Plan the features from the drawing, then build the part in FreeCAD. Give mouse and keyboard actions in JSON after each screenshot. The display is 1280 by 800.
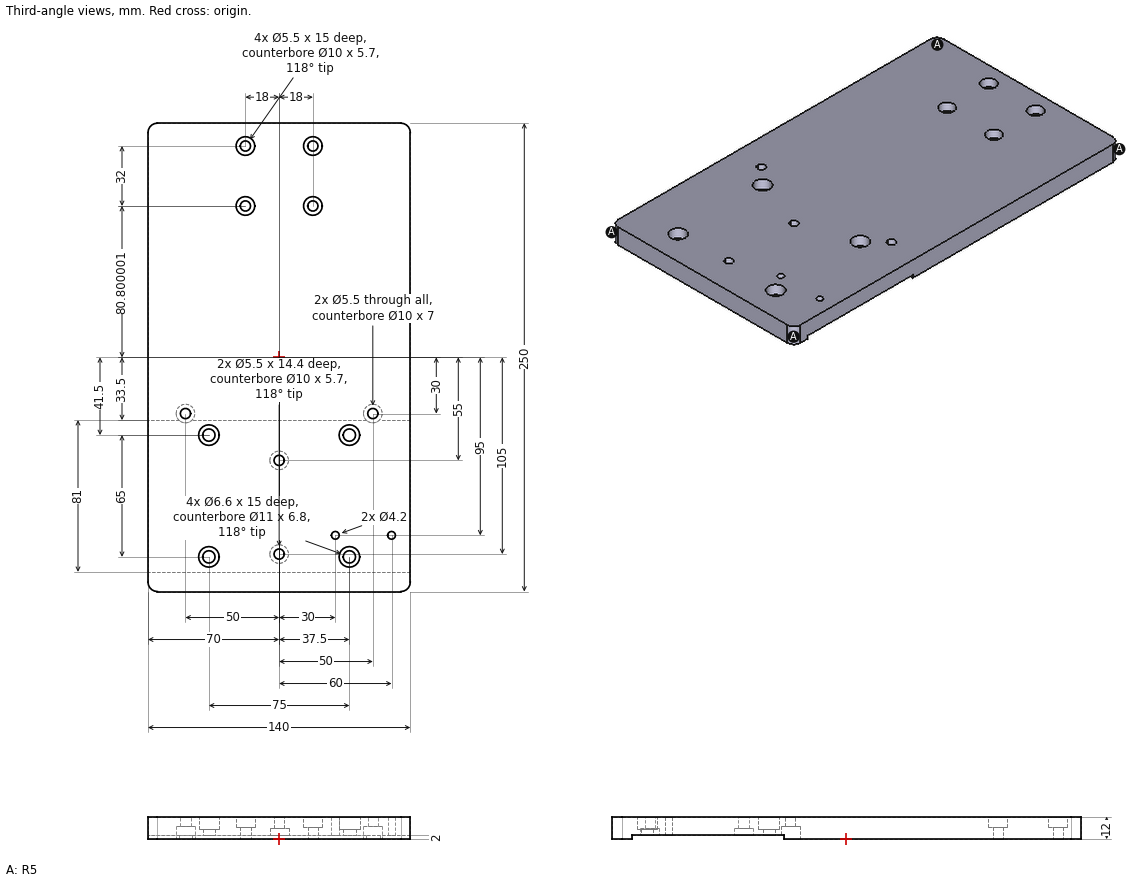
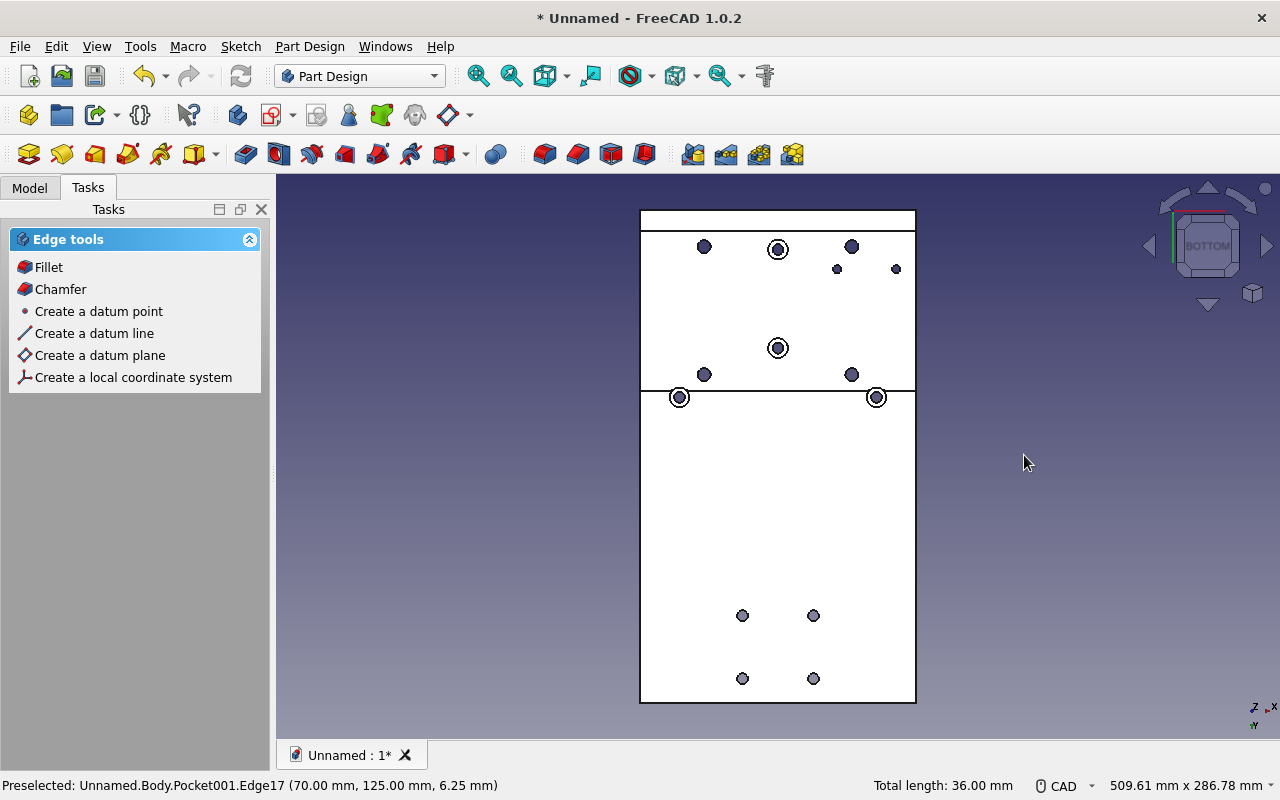
{"action": "key", "text": "4"}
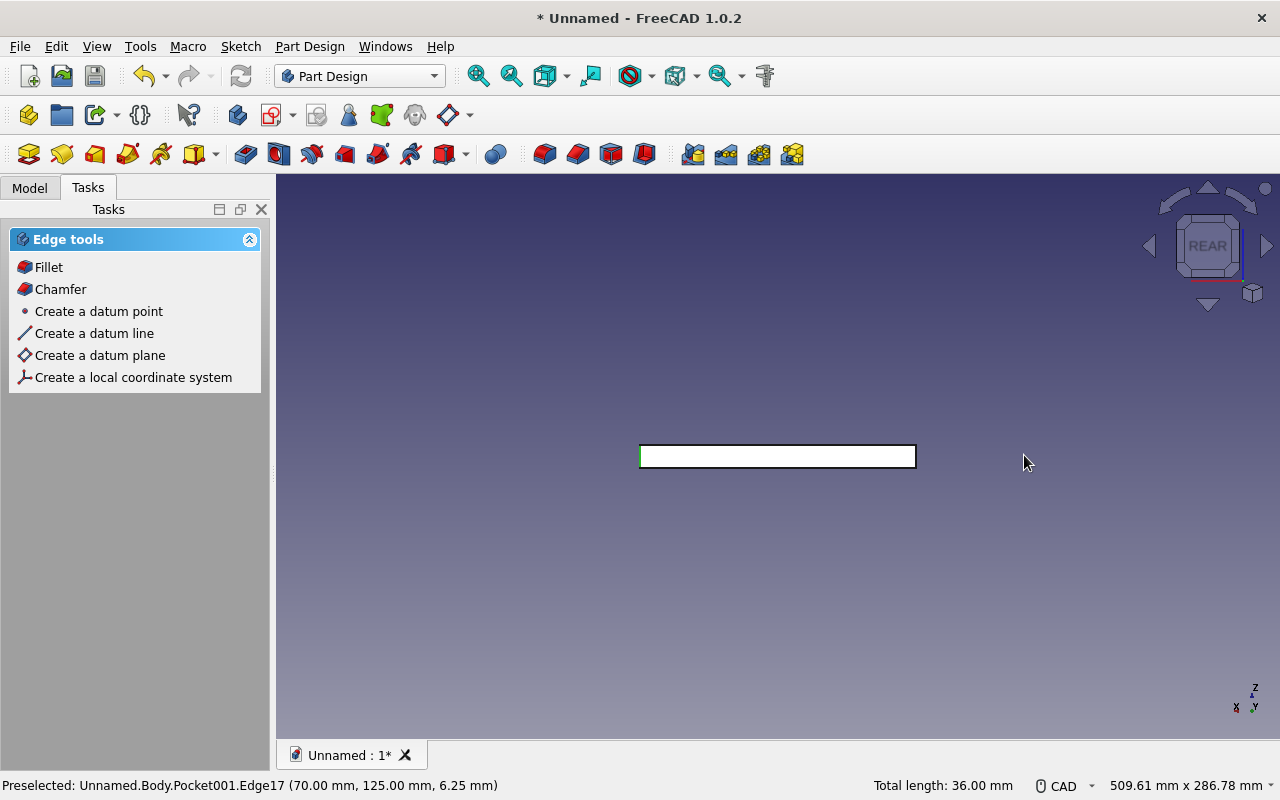
{"action": "left_click", "coordinate": [479, 76]}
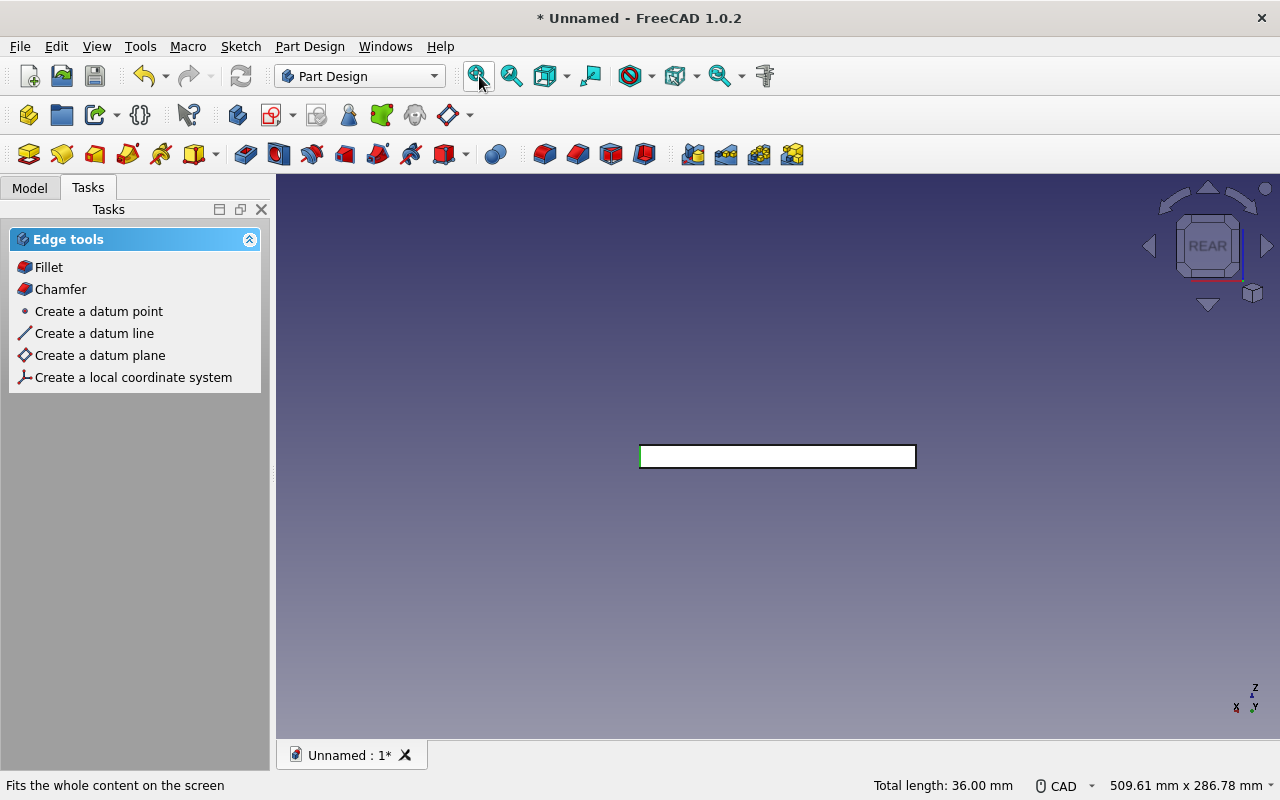
{"action": "left_click", "coordinate": [916, 456], "text": "ctrl"}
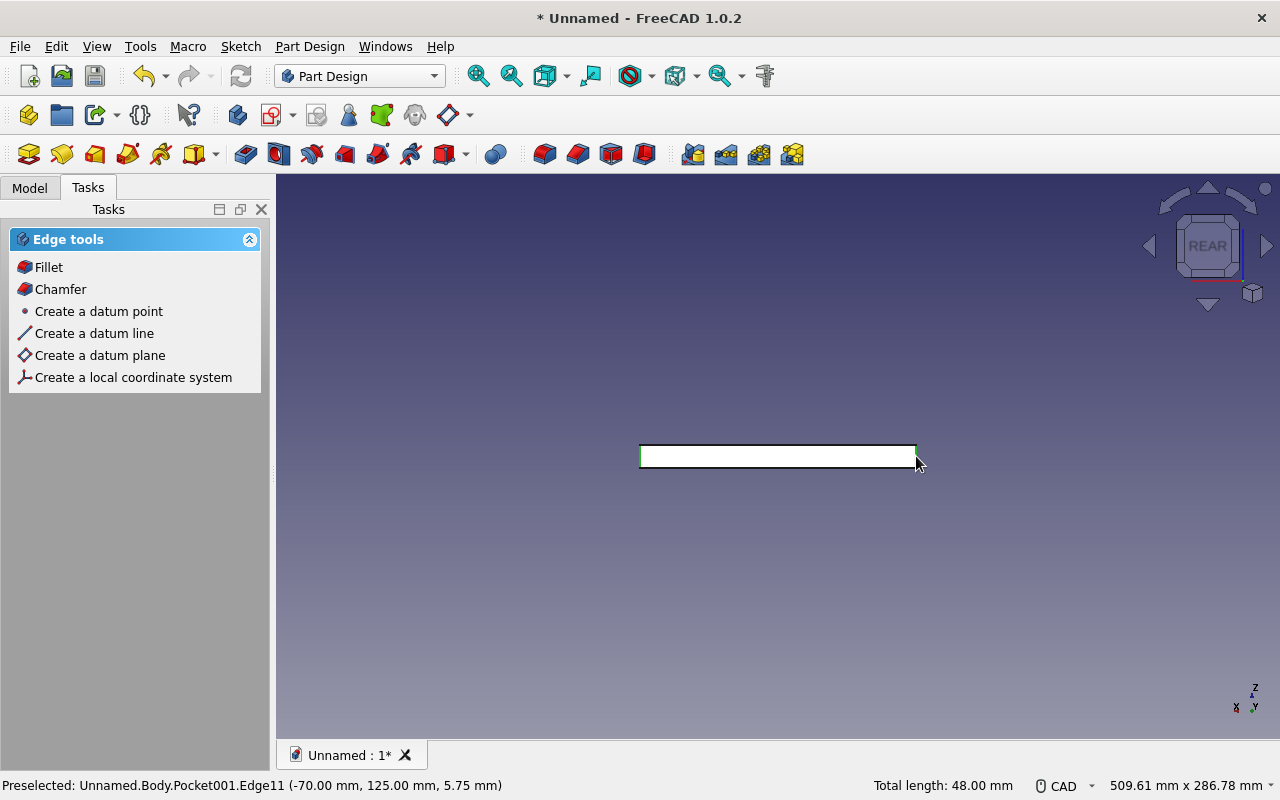
{"action": "left_click", "coordinate": [545, 154]}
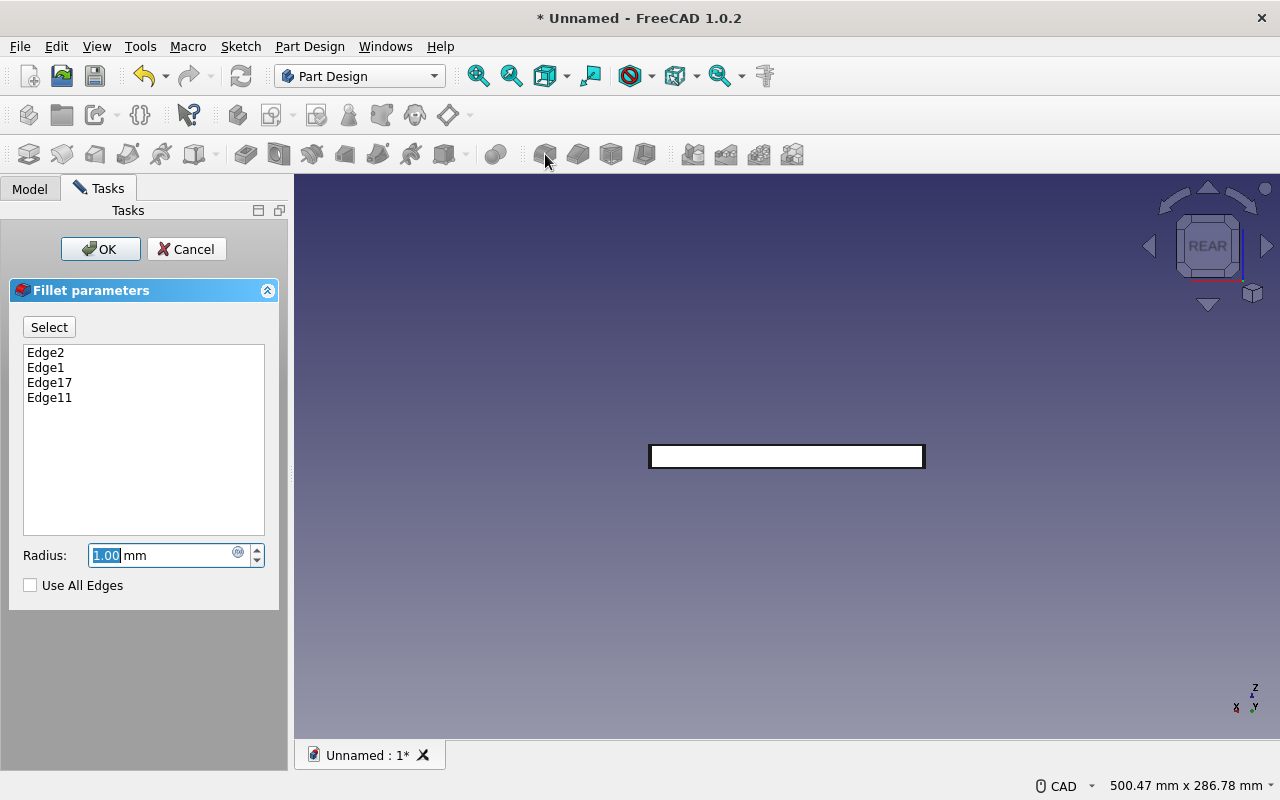
{"action": "type", "text": "5"}
{"action": "key", "text": "Tab"}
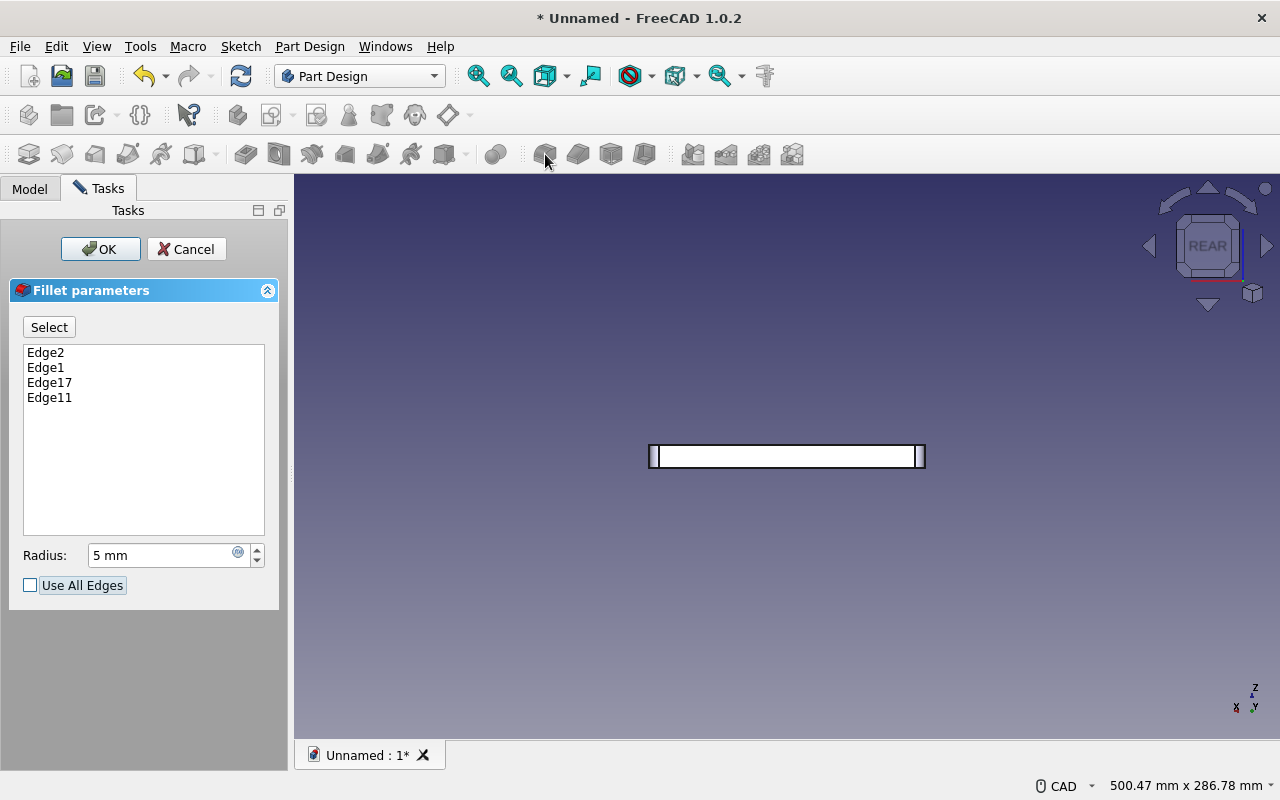
{"action": "left_click", "coordinate": [101, 249]}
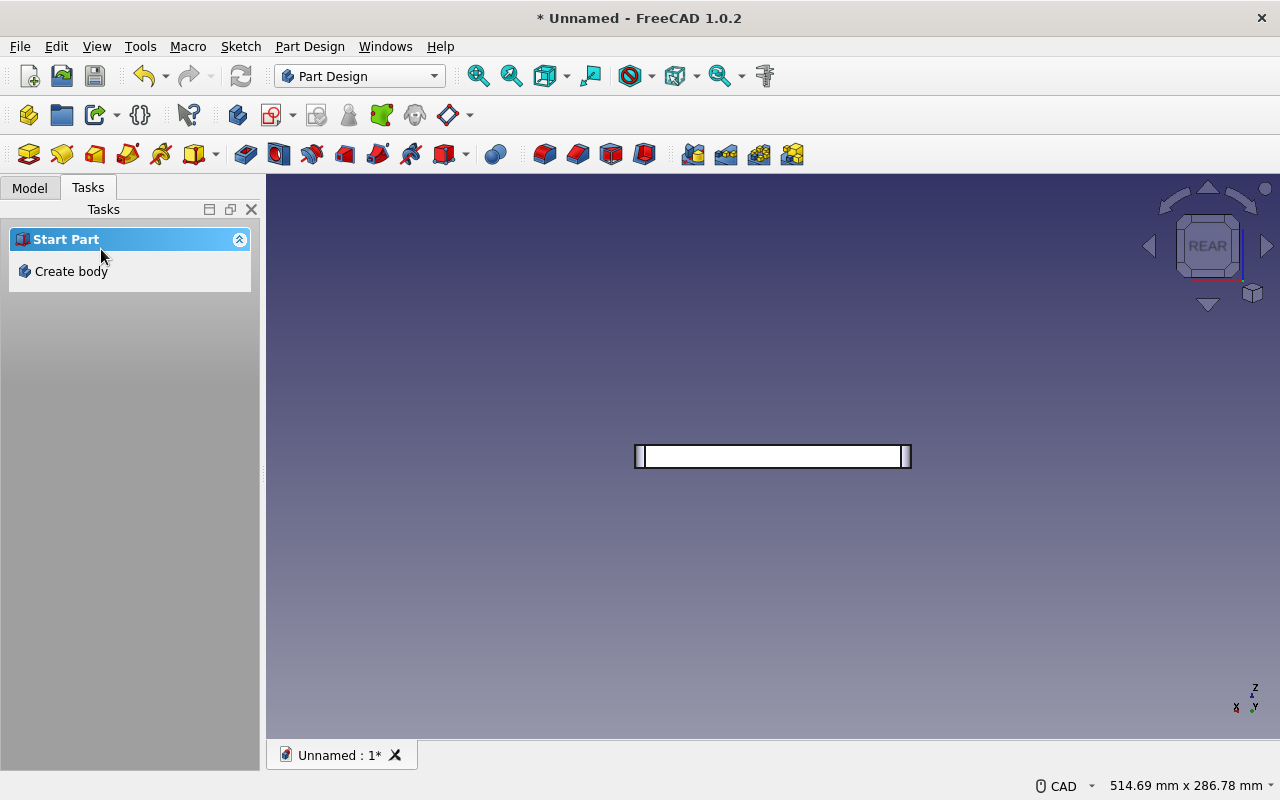
{"action": "key", "text": "0"}